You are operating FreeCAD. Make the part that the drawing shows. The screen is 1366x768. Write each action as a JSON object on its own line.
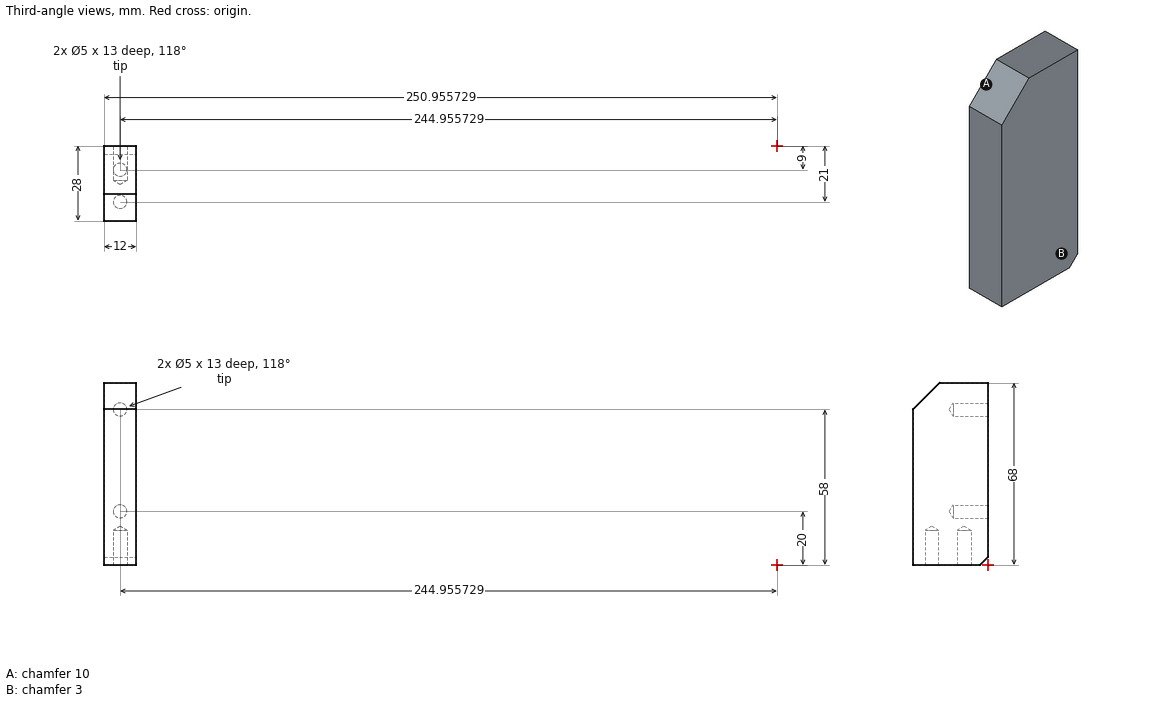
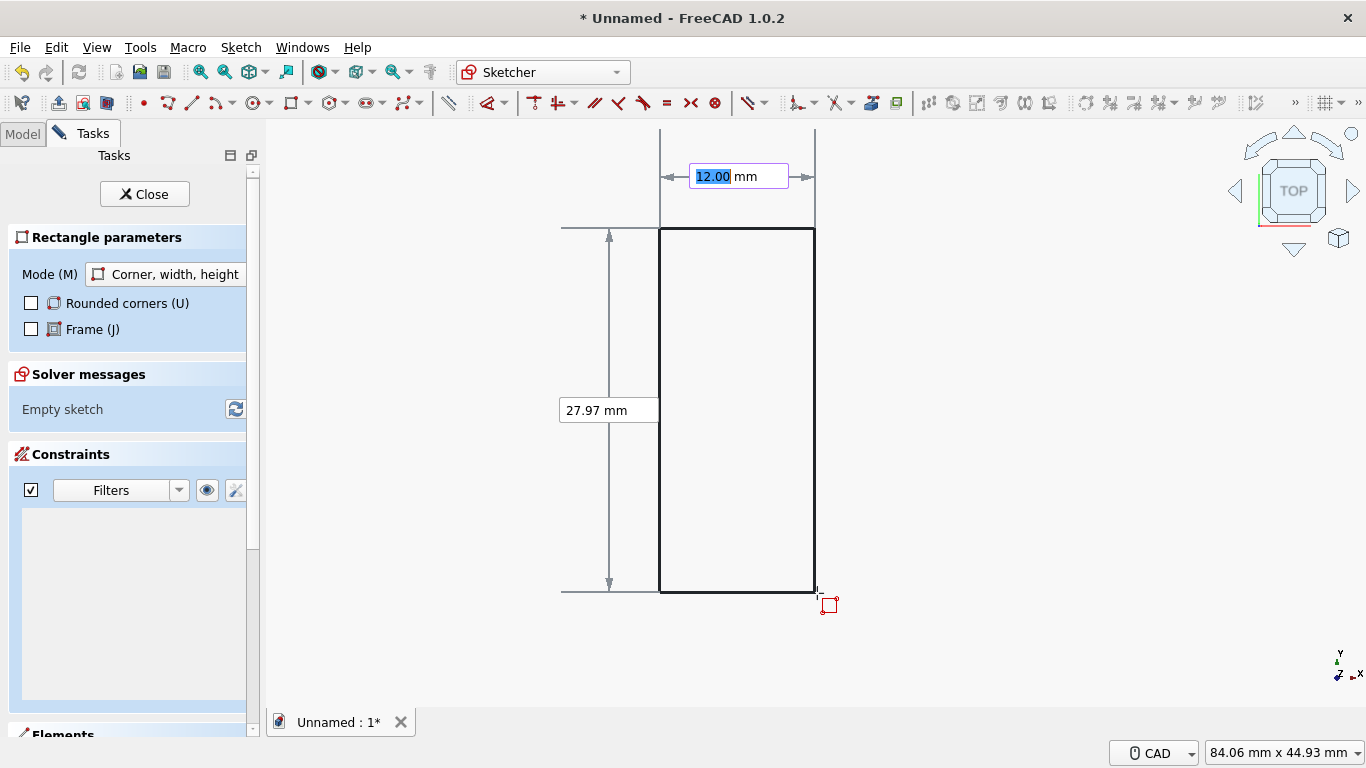
{"action": "type", "text": "12"}
{"action": "key", "text": "Tab"}
{"action": "type", "text": "28"}
{"action": "key", "text": "Return"}
{"action": "key", "text": "Escape"}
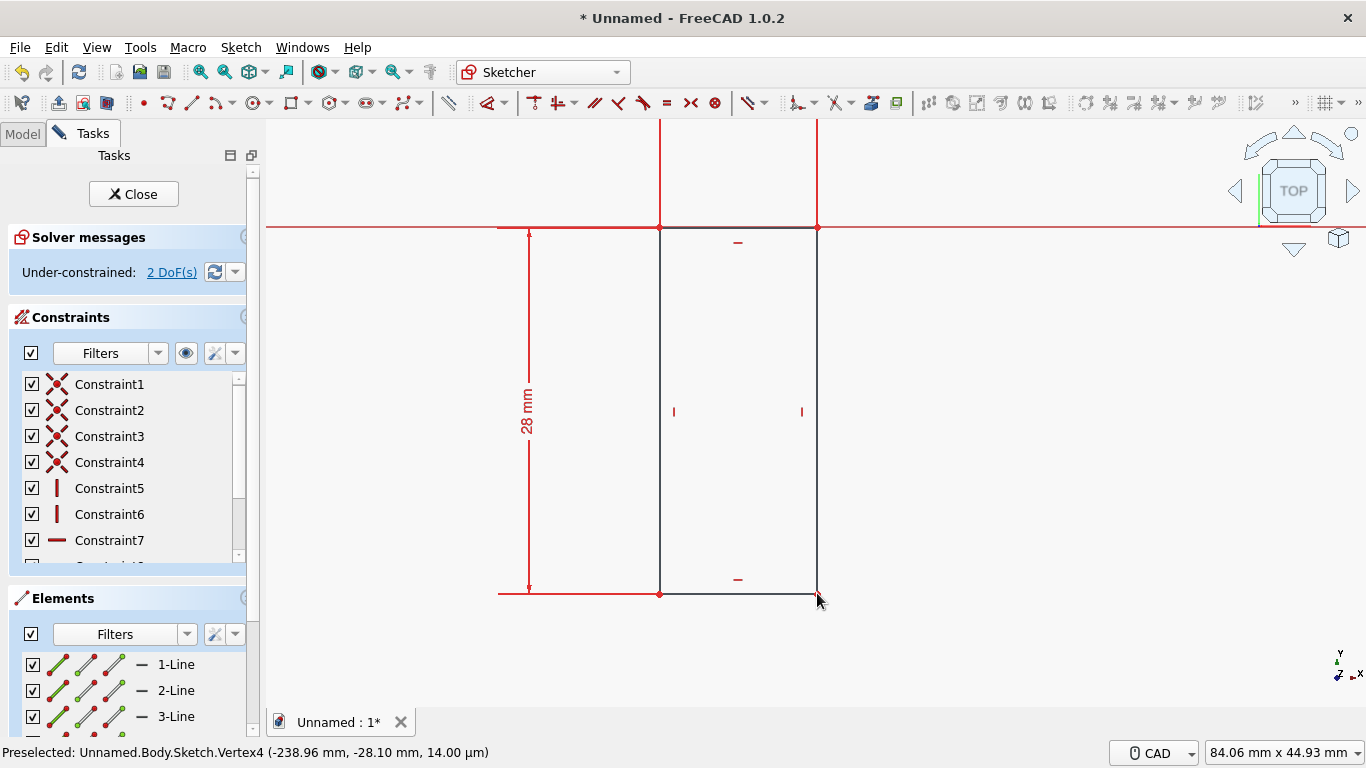
{"action": "left_click", "coordinate": [660, 228]}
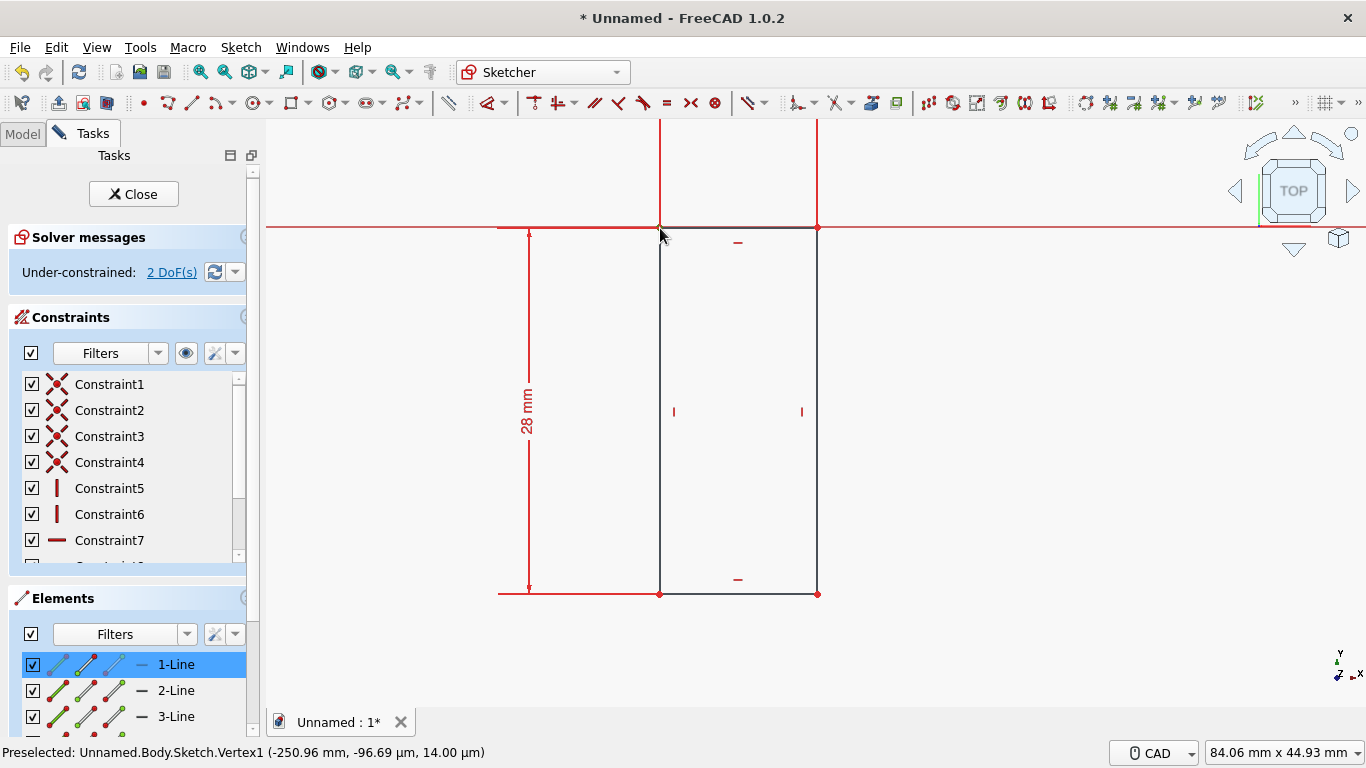
{"action": "left_click", "coordinate": [359, 227]}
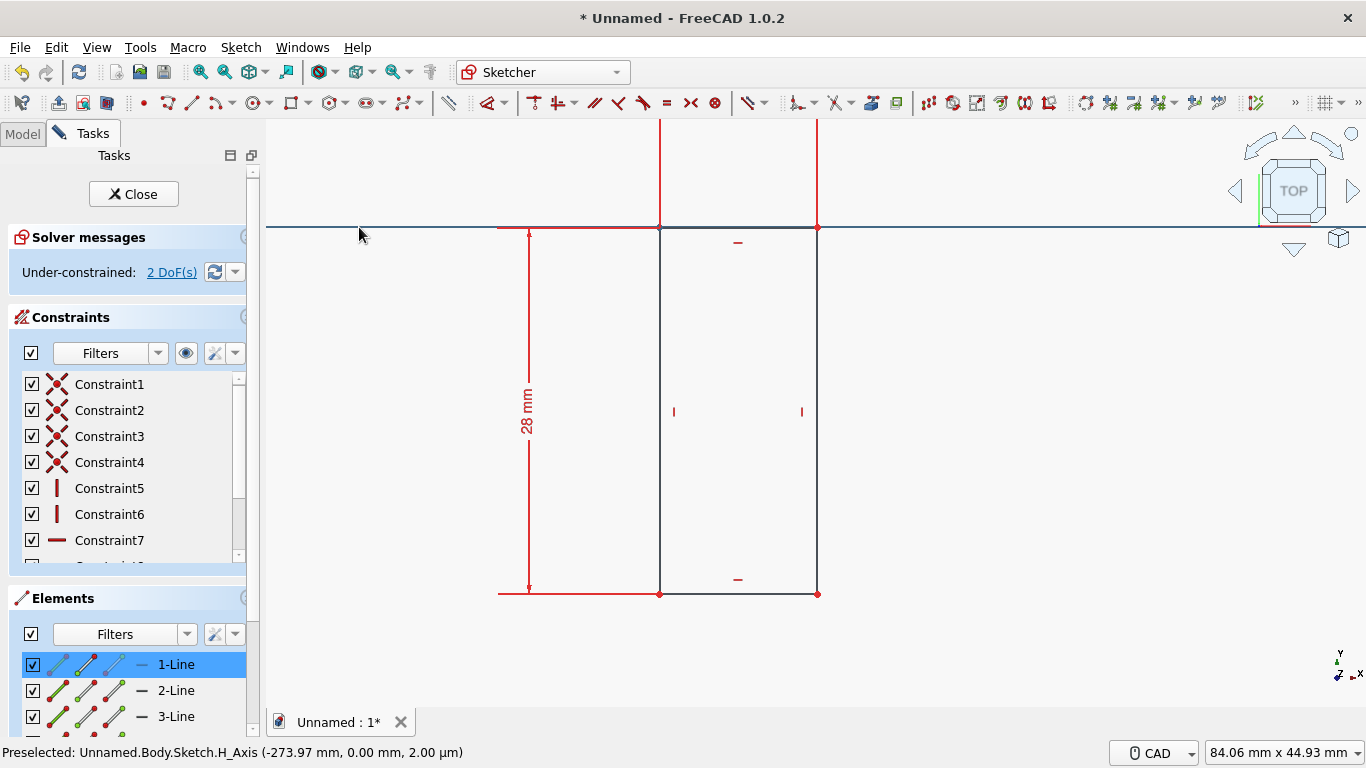
{"action": "key", "text": "c"}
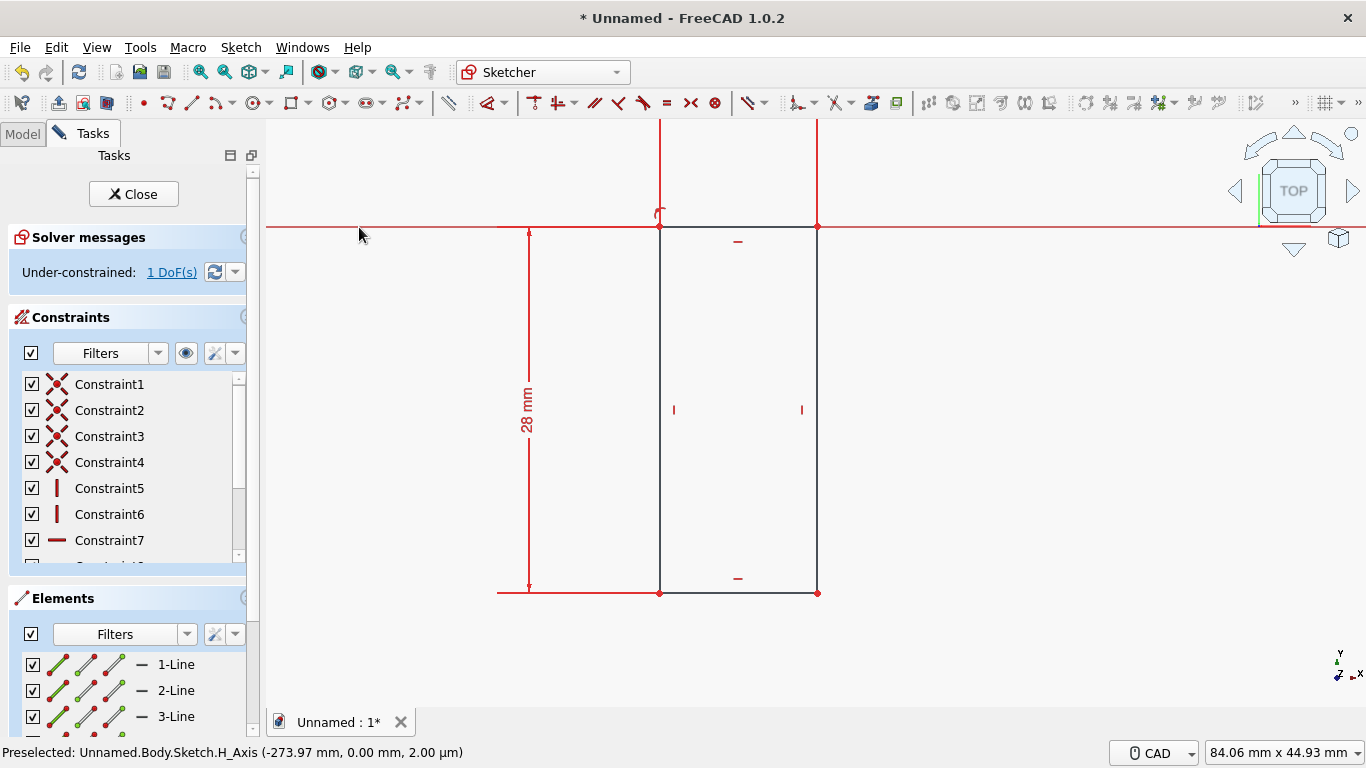
{"action": "left_click", "coordinate": [488, 104]}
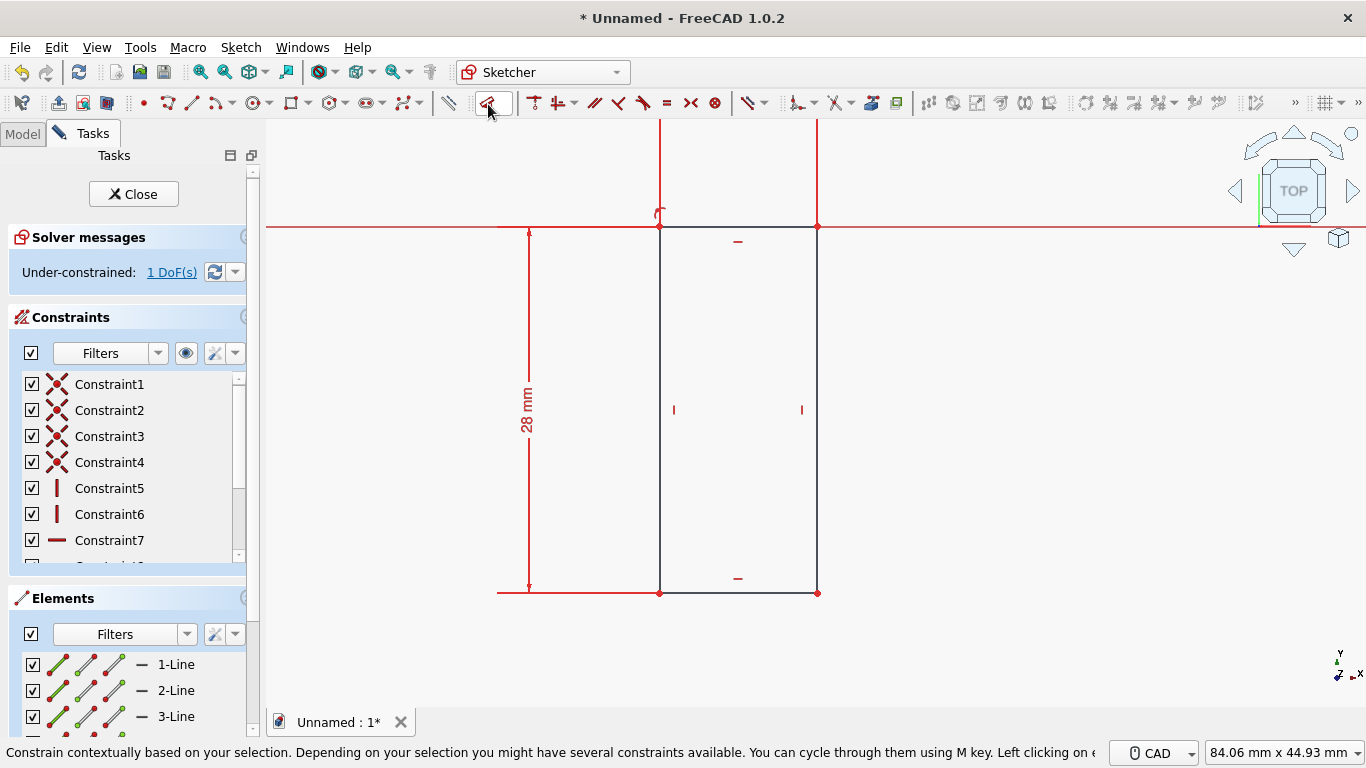
{"action": "left_click", "coordinate": [660, 227]}
{"action": "left_click", "coordinate": [930, 193]}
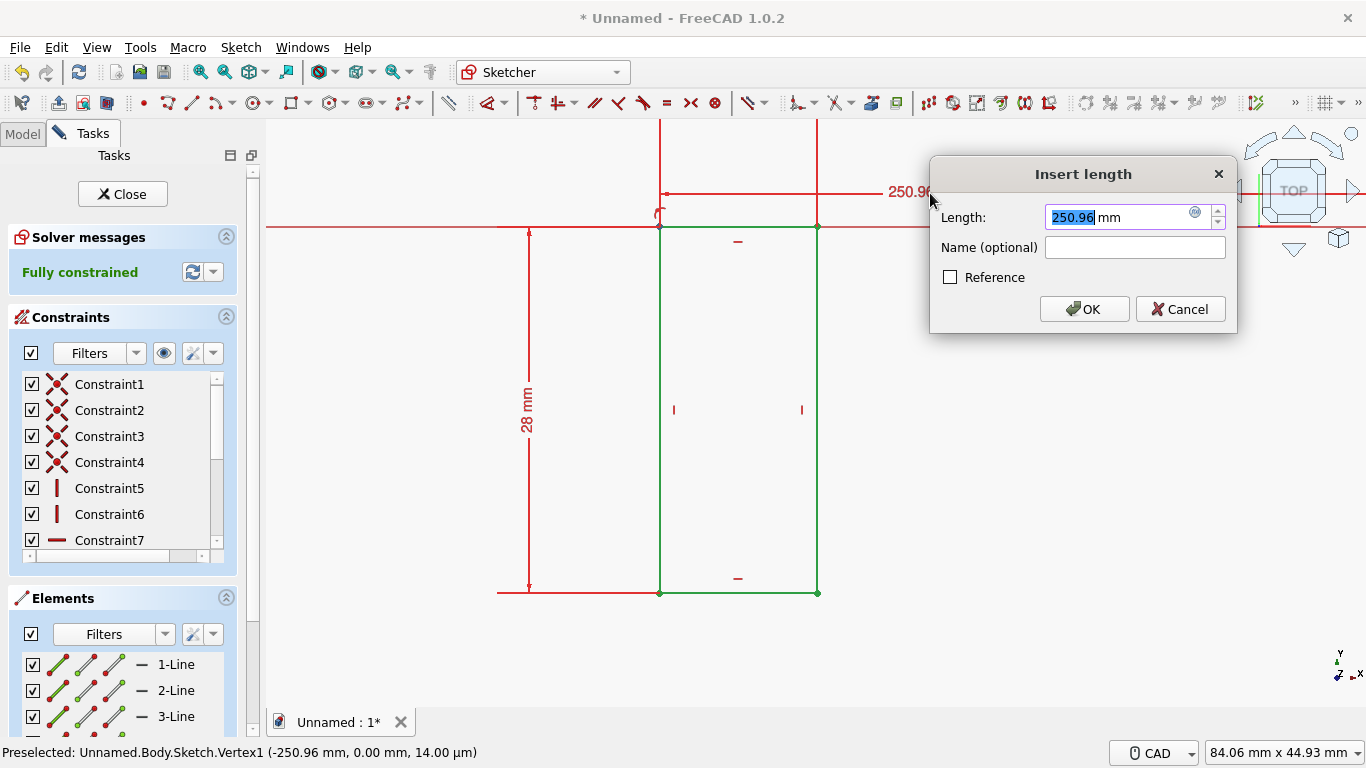
{"action": "type", "text": "250.955729"}
{"action": "key", "text": "Return"}
{"action": "key", "text": "Escape"}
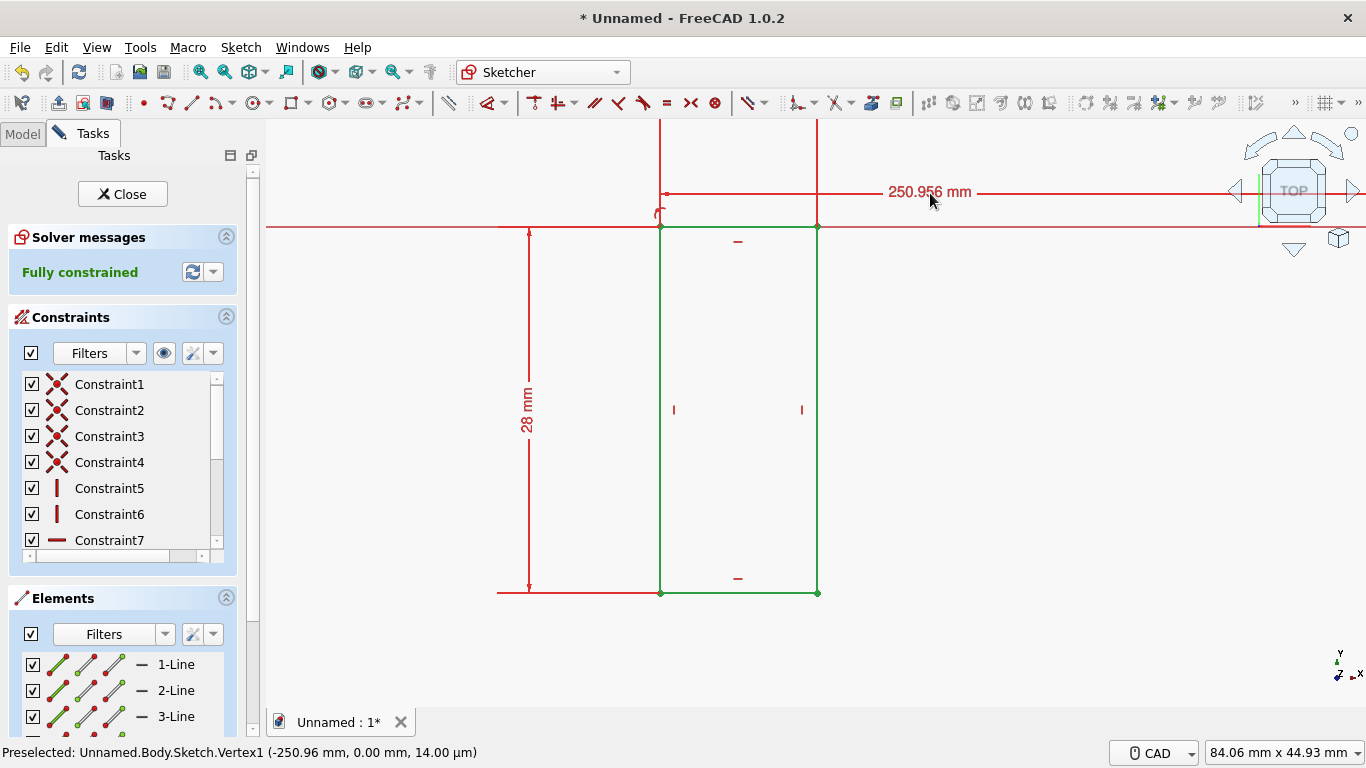
{"action": "left_click", "coordinate": [123, 194]}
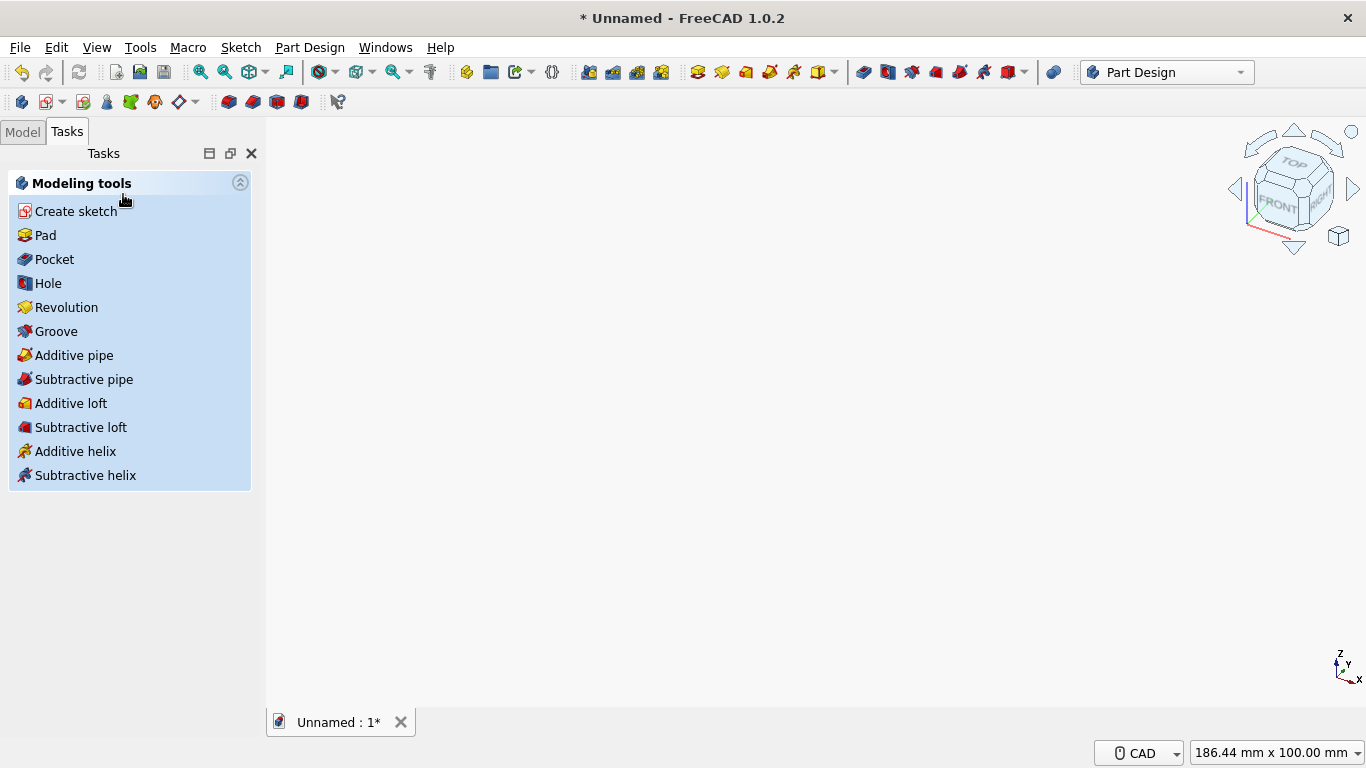
{"action": "left_click", "coordinate": [698, 72]}